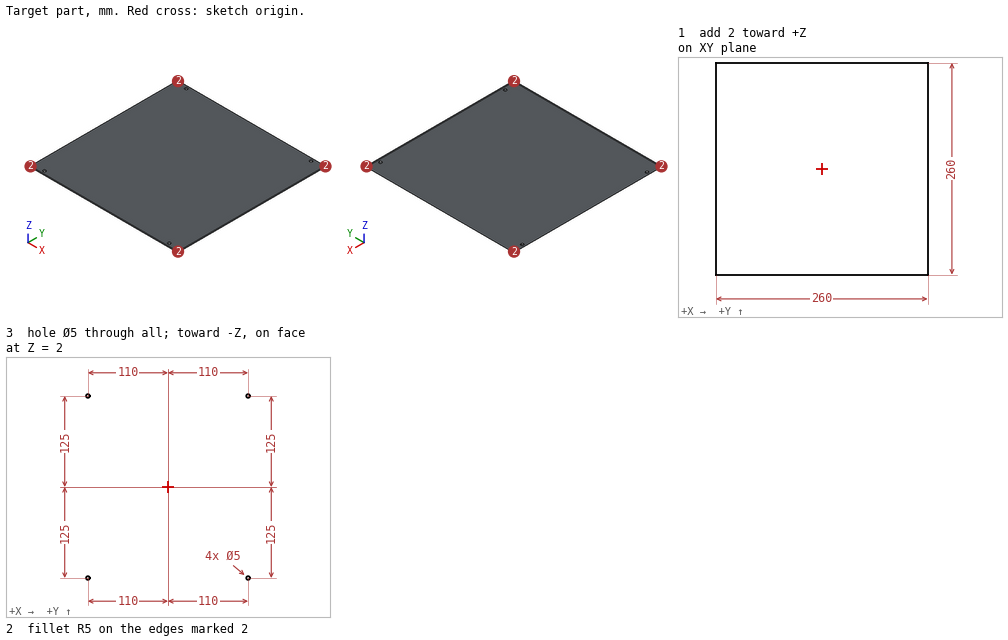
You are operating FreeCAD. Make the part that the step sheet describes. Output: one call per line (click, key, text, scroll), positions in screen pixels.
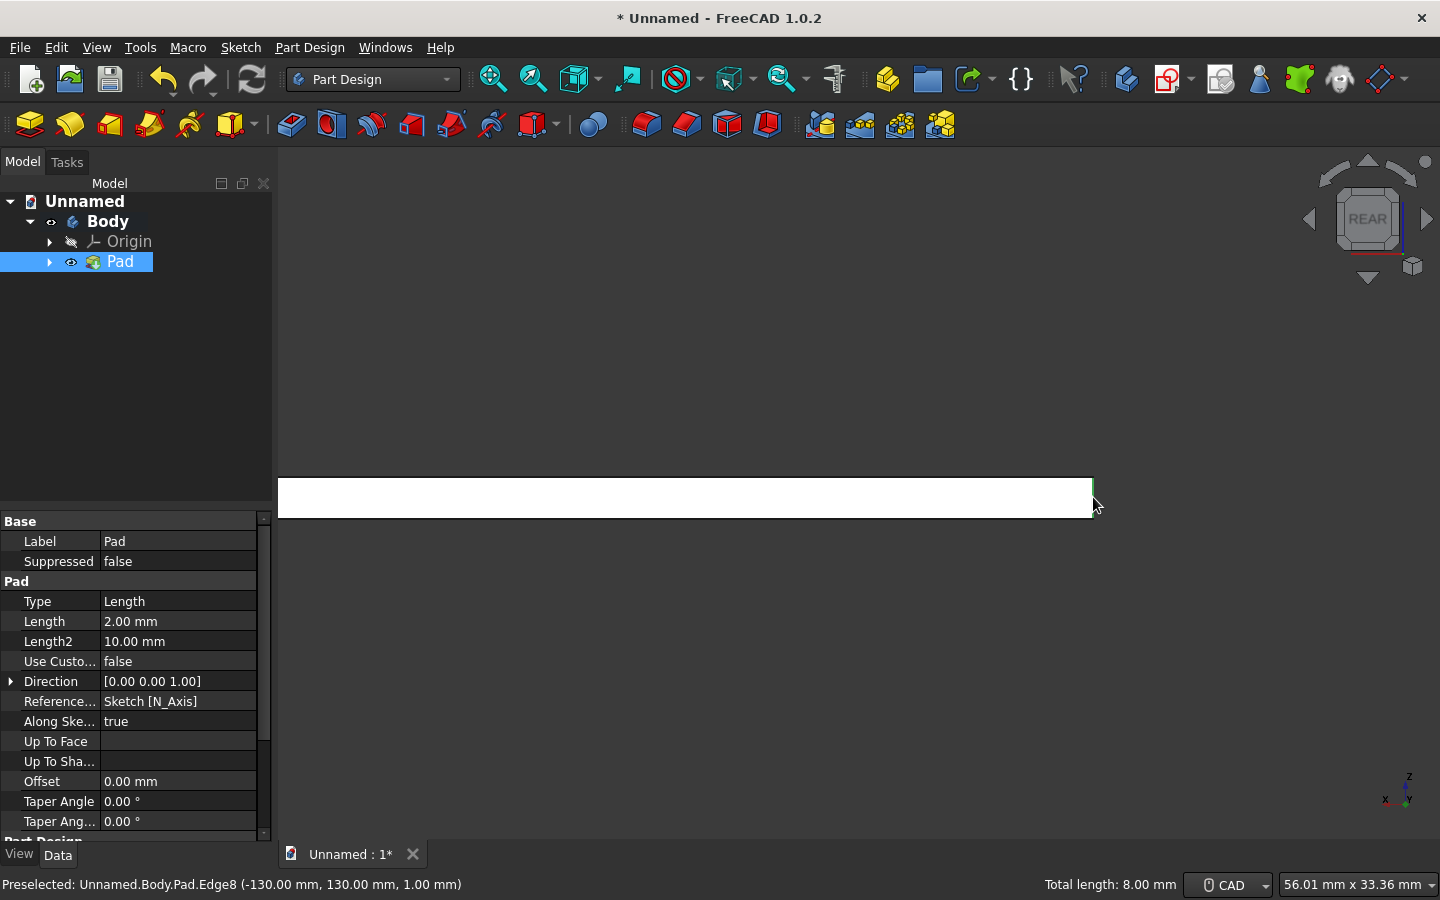
click(648, 124)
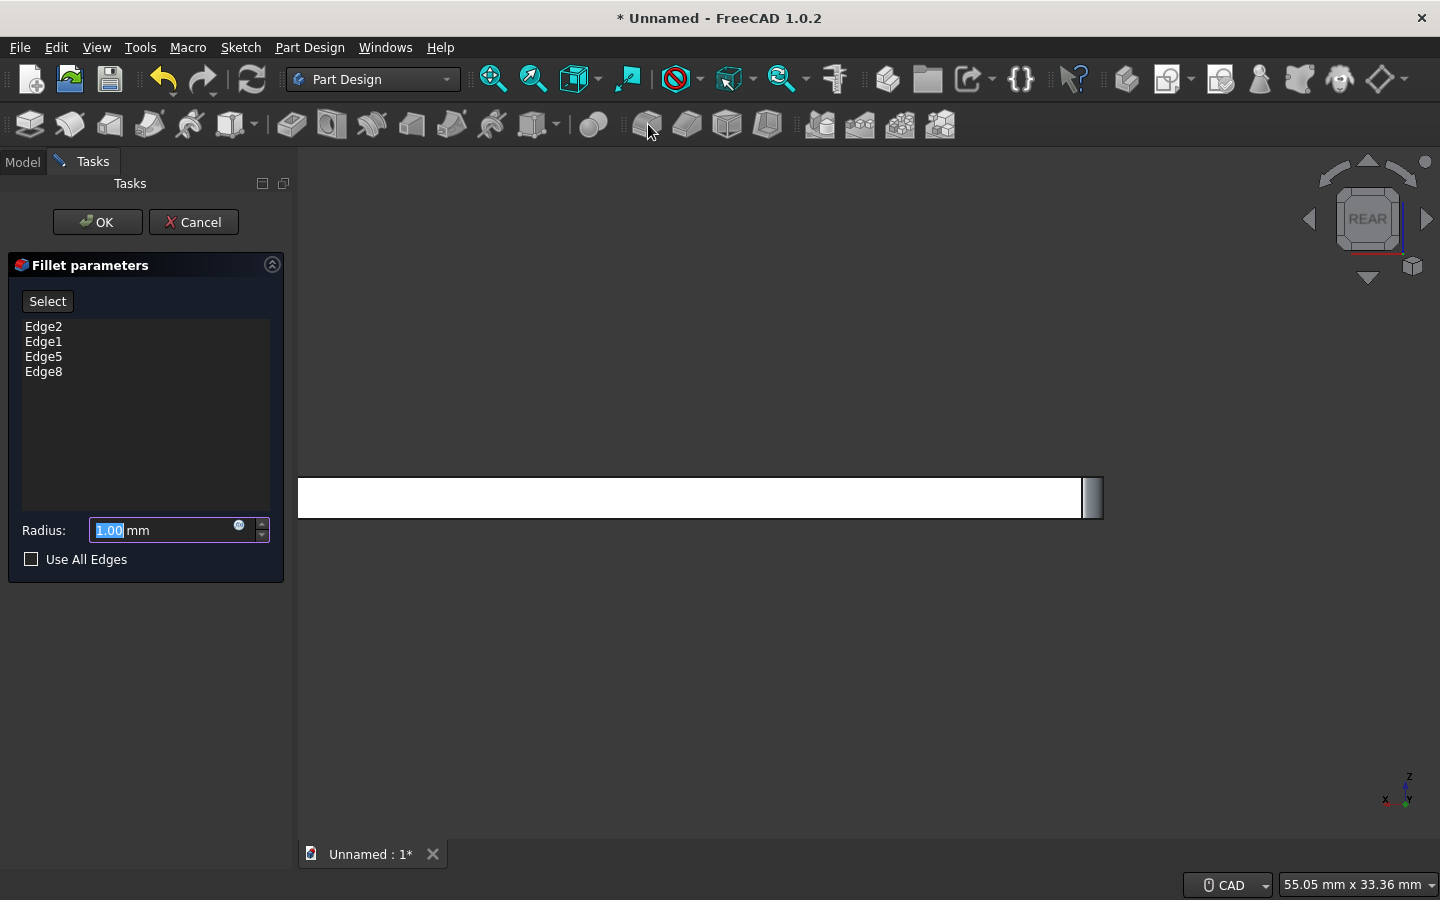
text(5)
key(Tab)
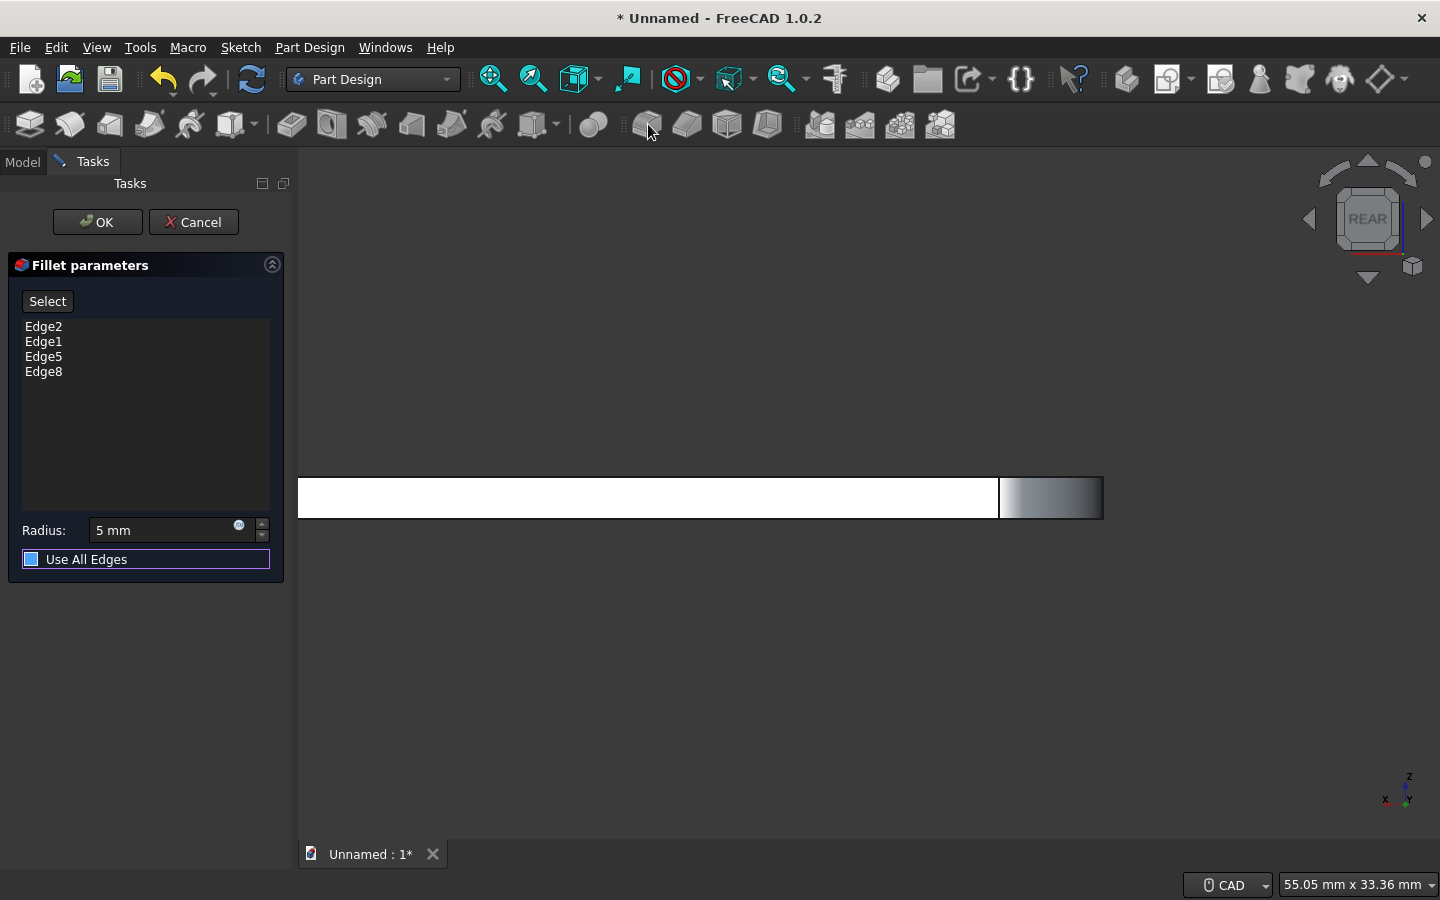
click(98, 222)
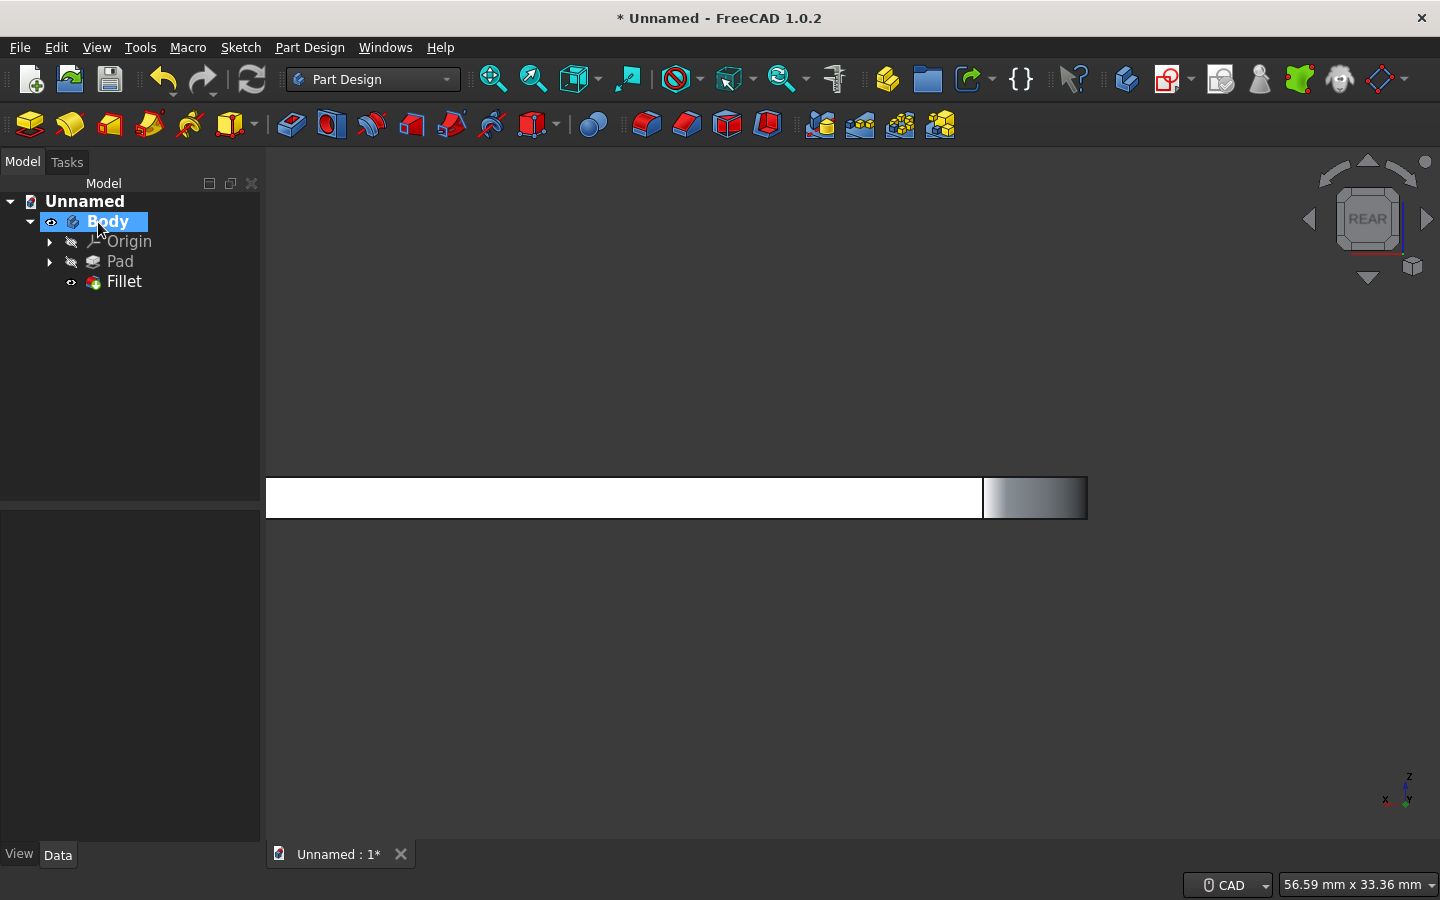
click(494, 80)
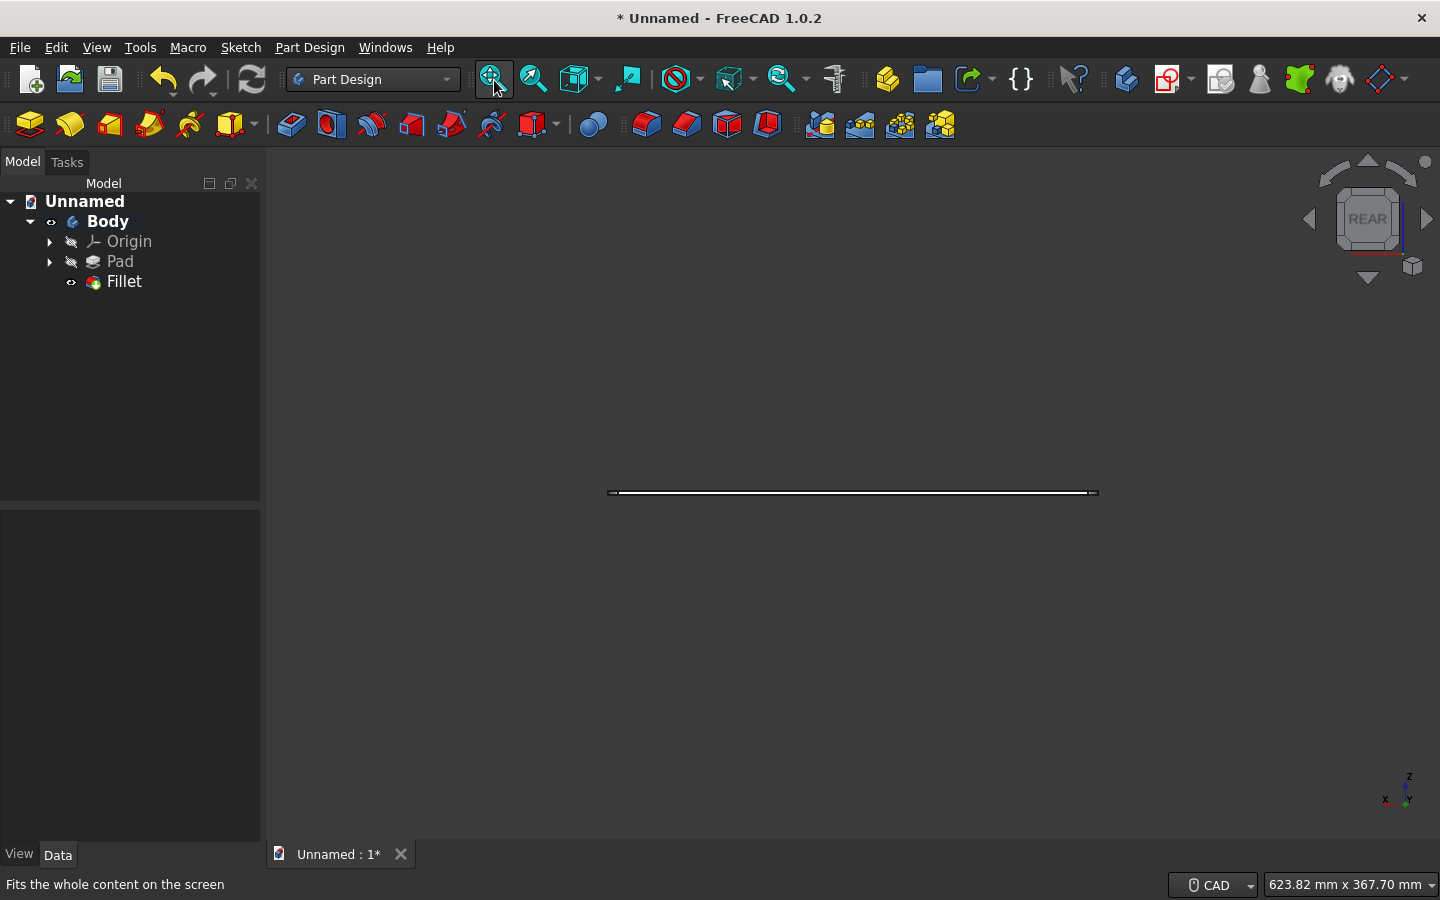
key(0)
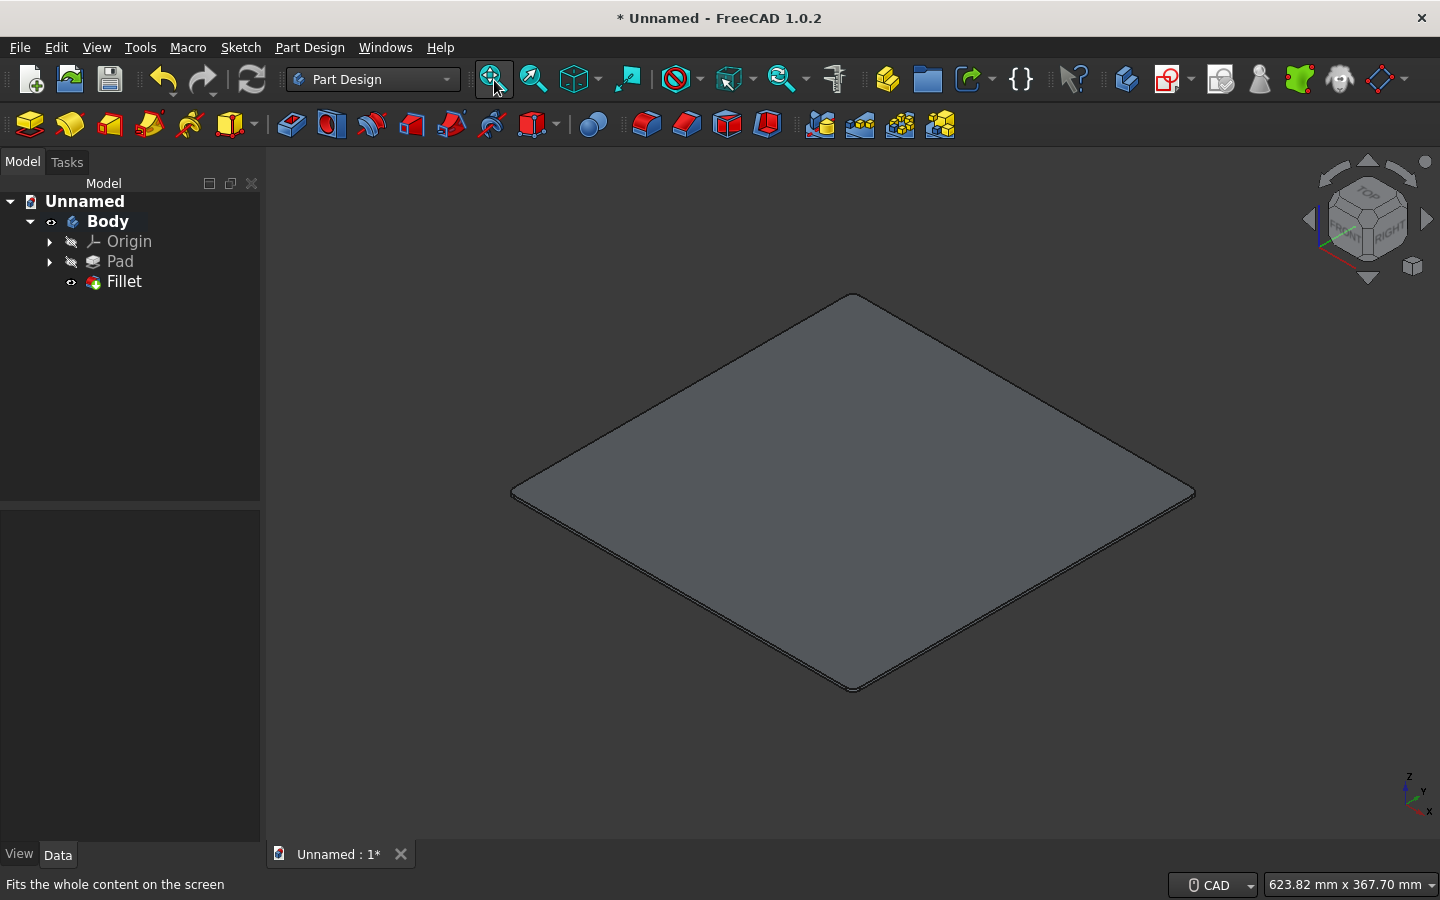
click(853, 490)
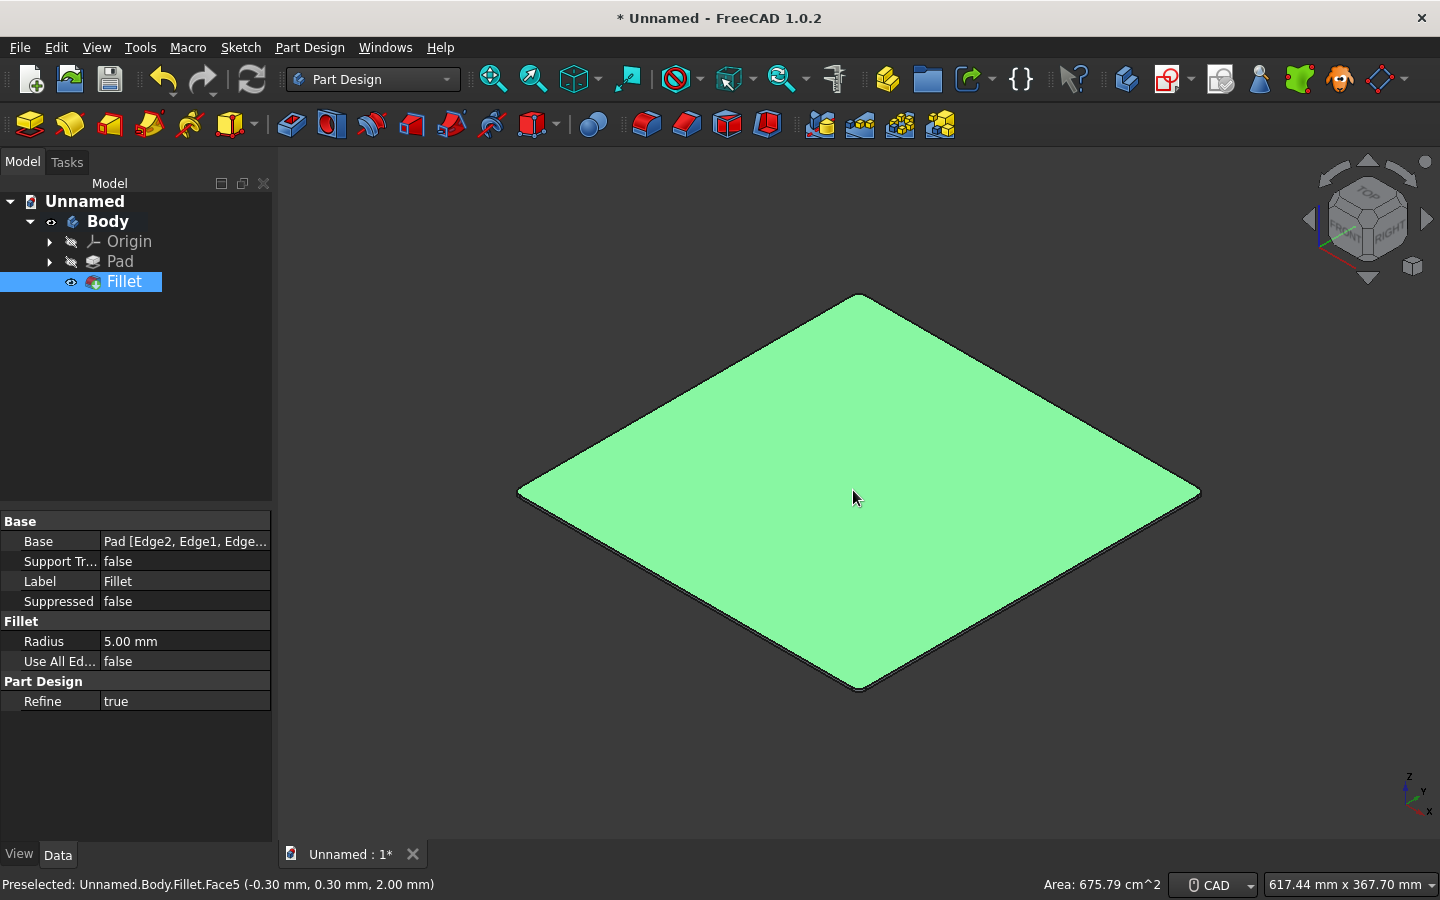
click(1168, 80)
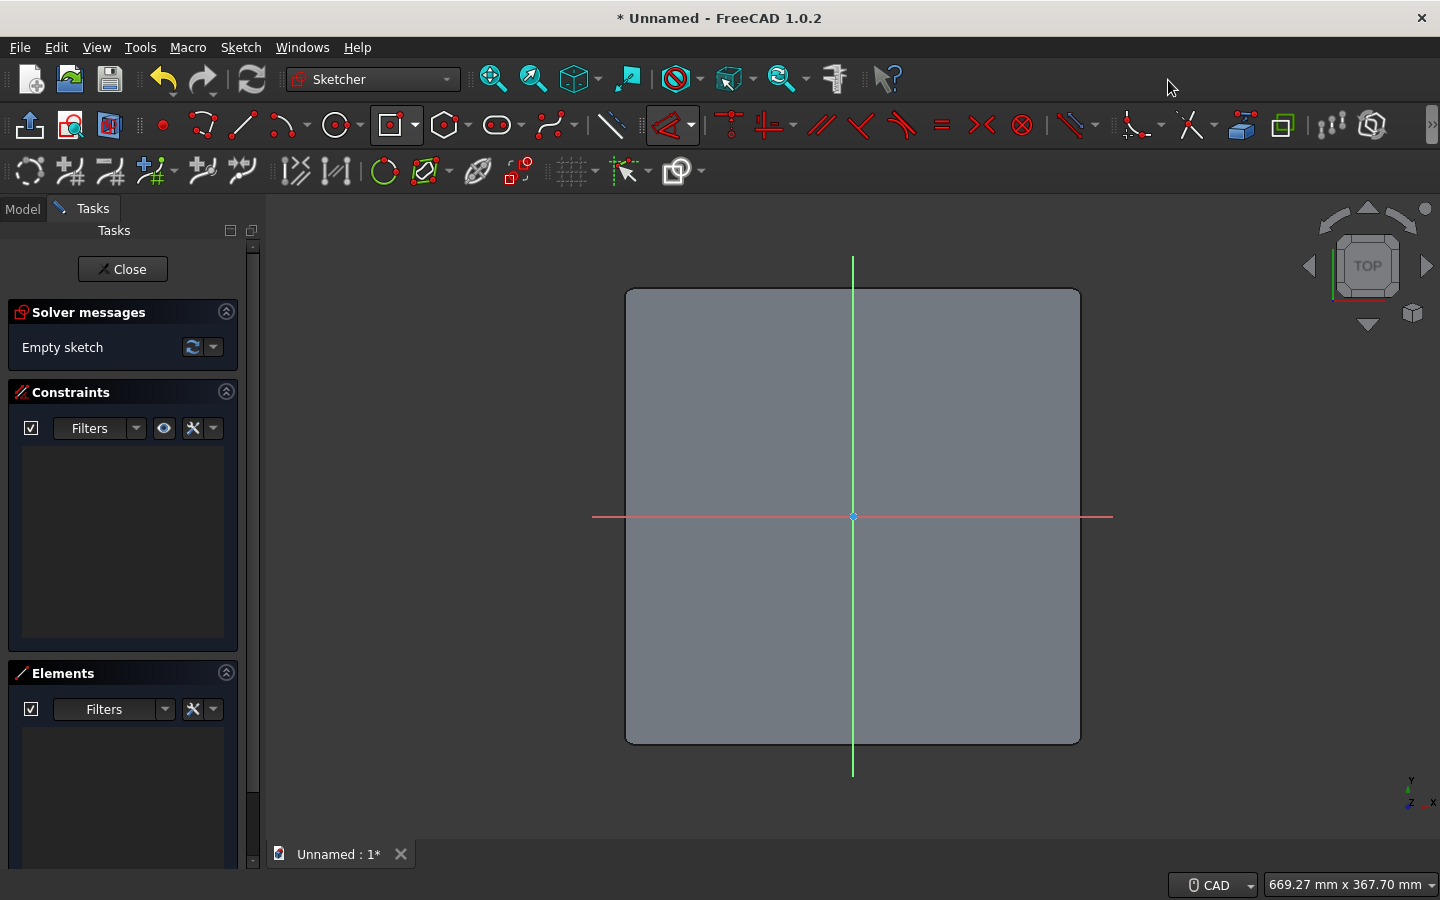
key(g)
key(c)